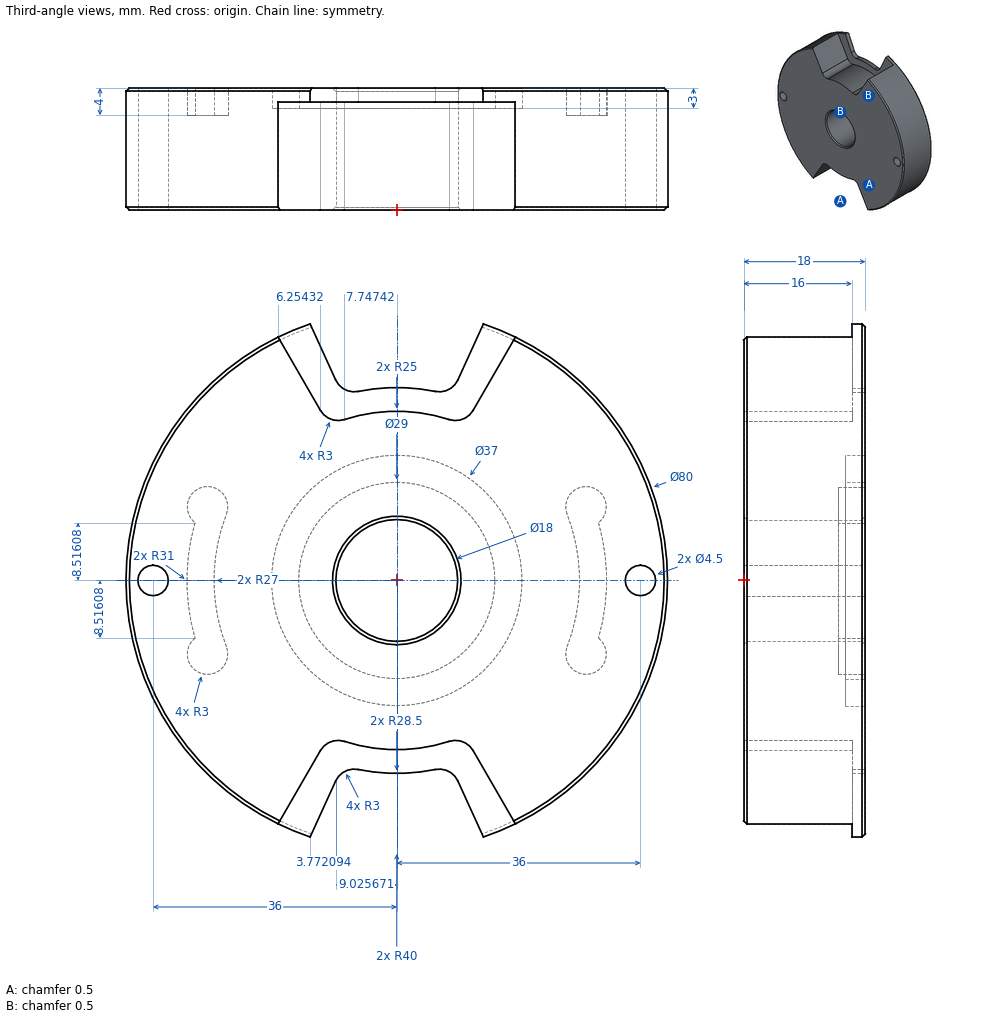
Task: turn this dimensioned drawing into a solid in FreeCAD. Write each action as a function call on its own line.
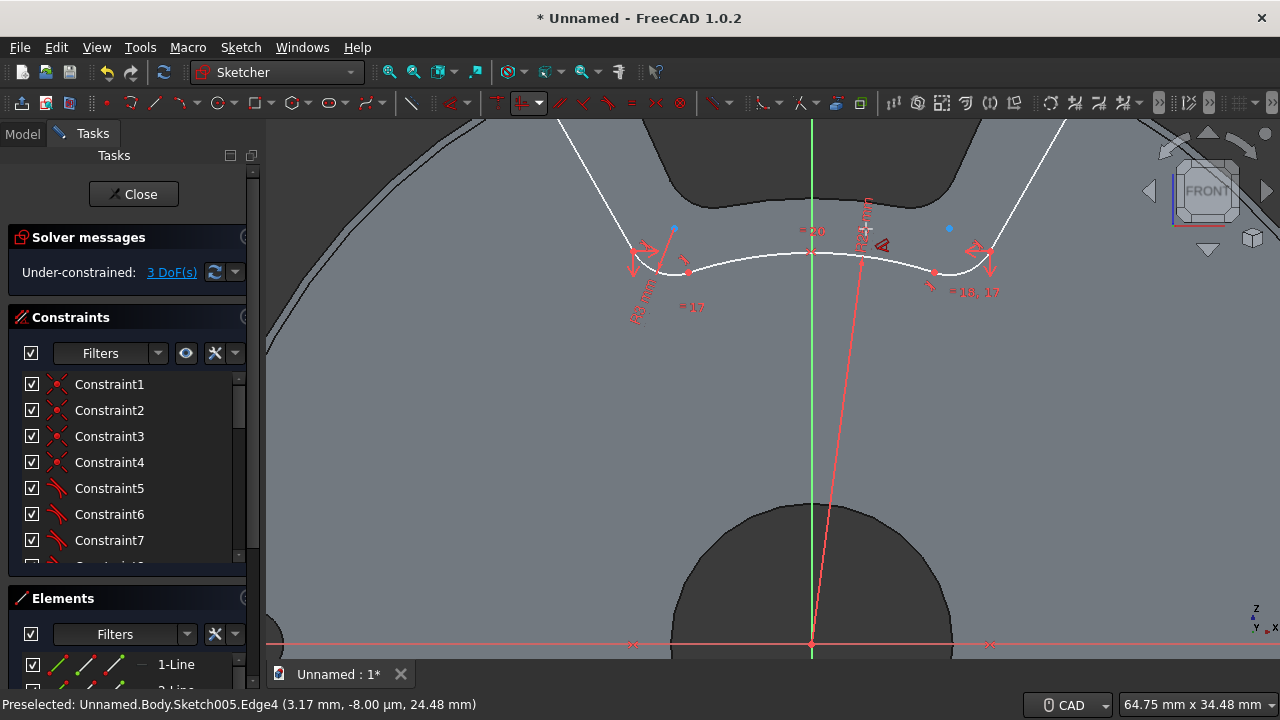
scroll(658, 279, down, 6)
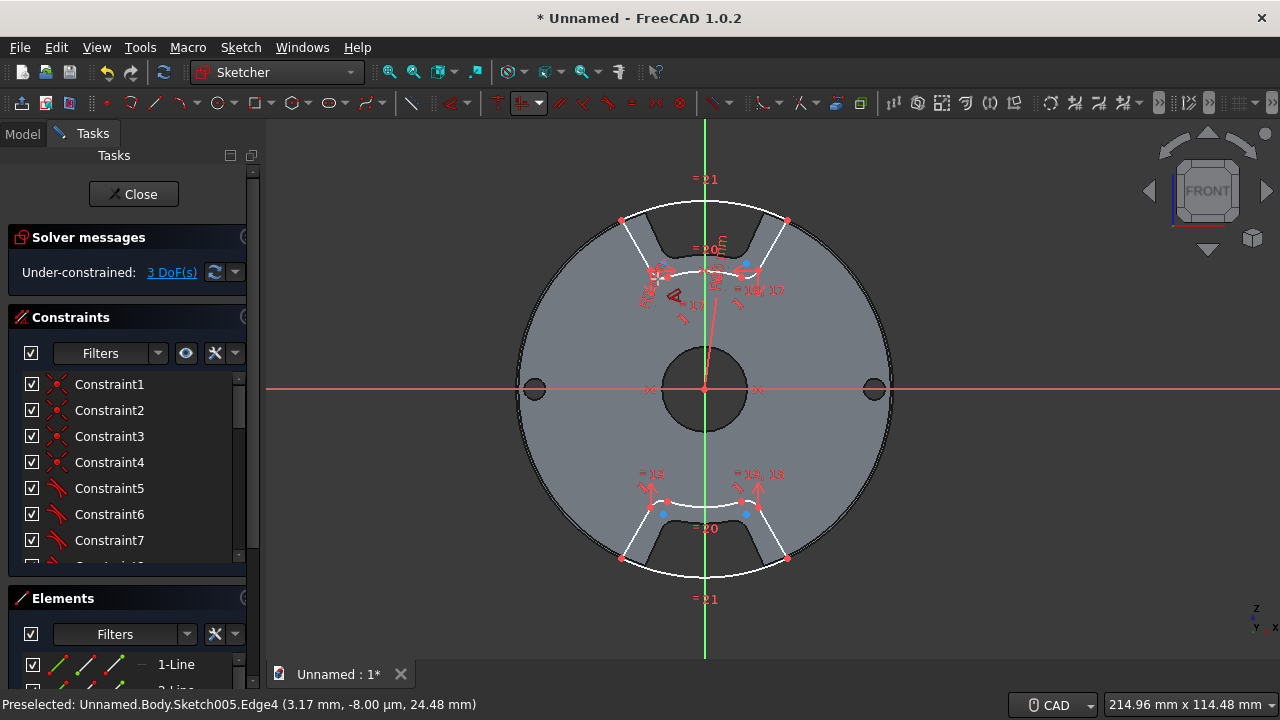
click(739, 204)
click(745, 173)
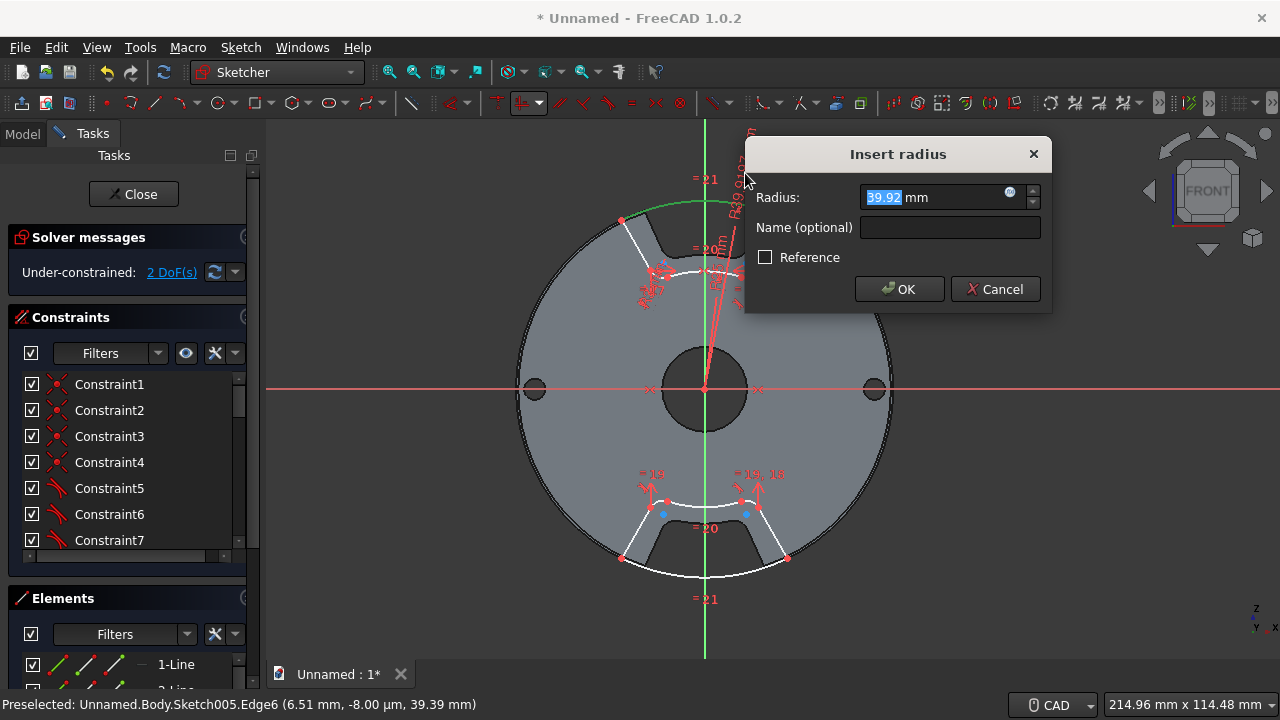
text(40)
key(Return)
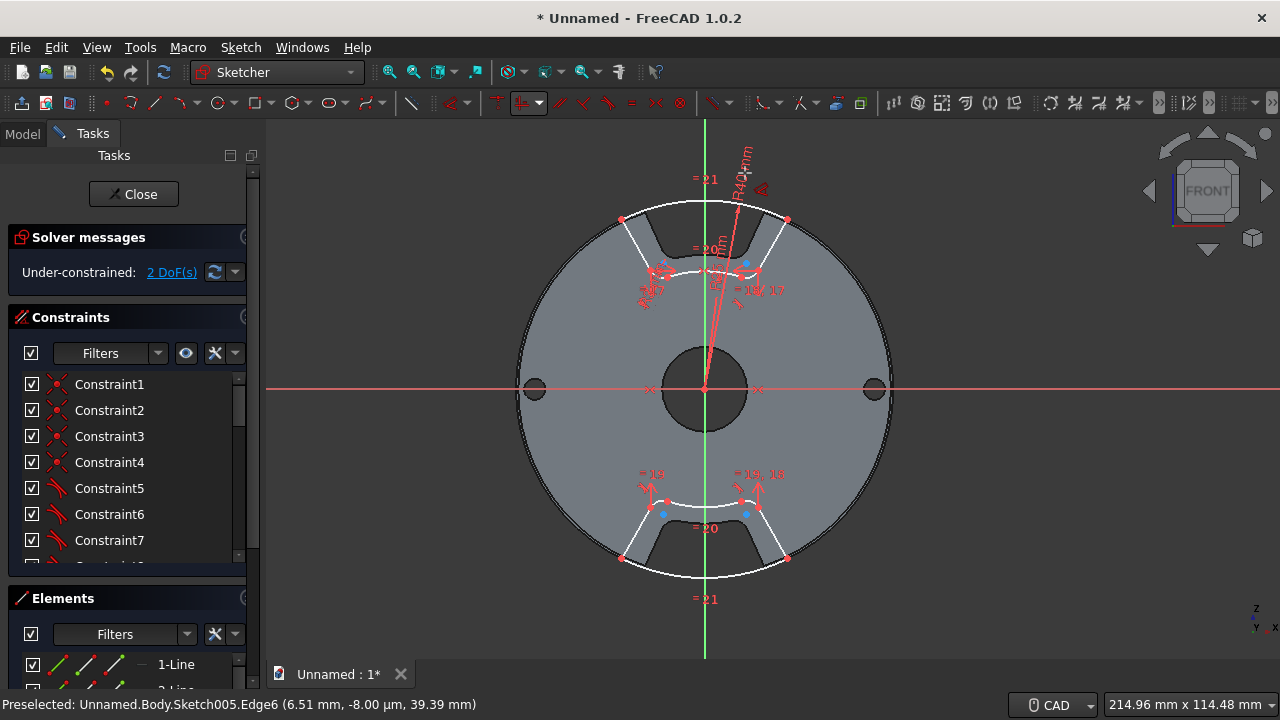
click(668, 277)
click(686, 243)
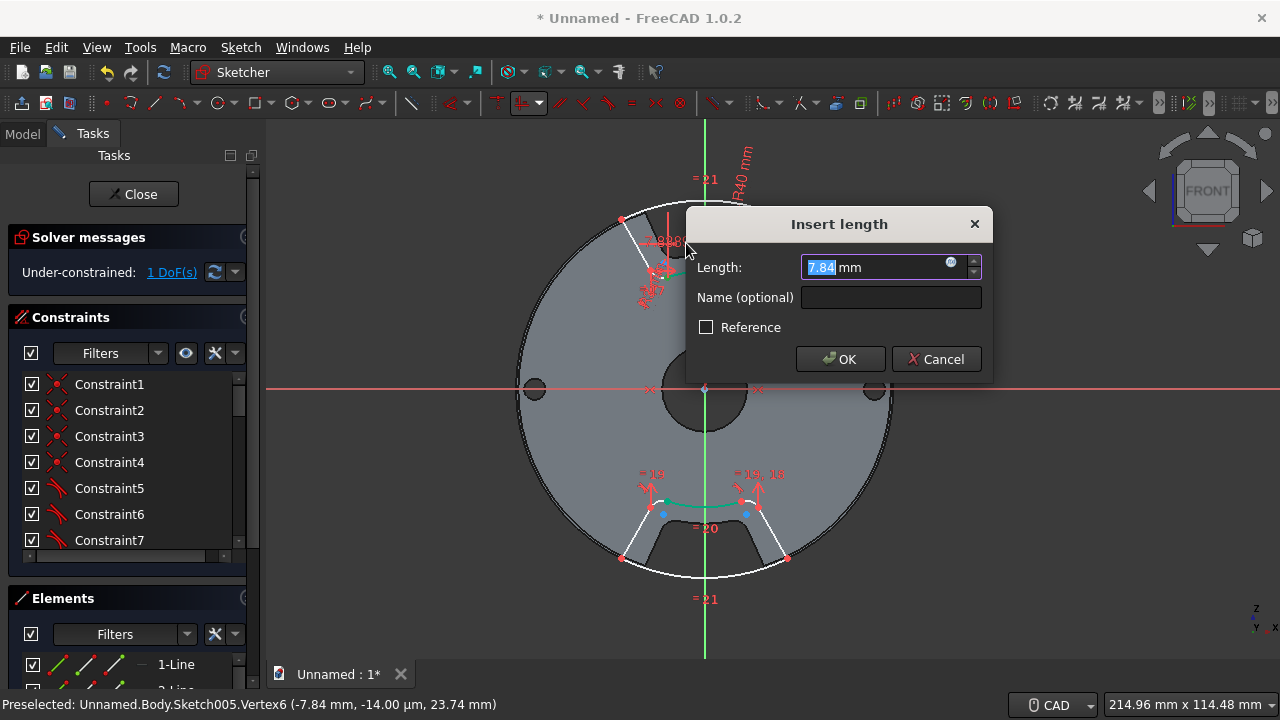
text(7.74742)
key(Return)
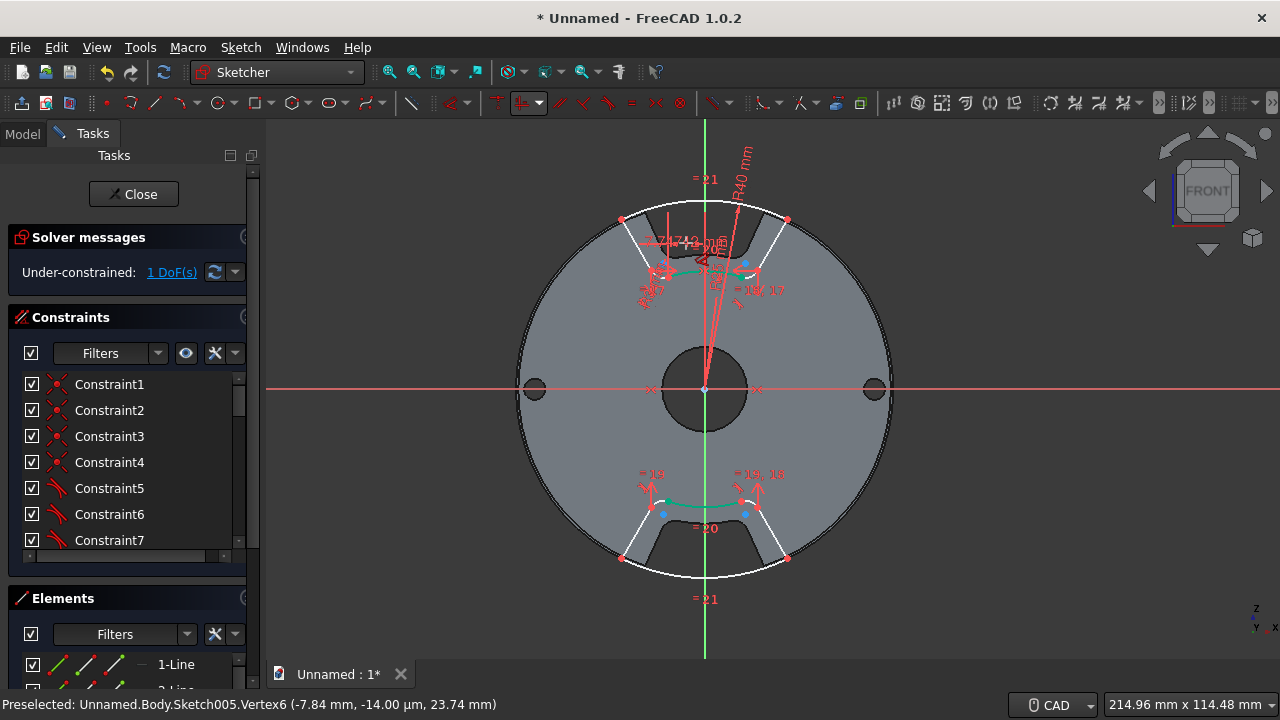
scroll(631, 235, up, 2)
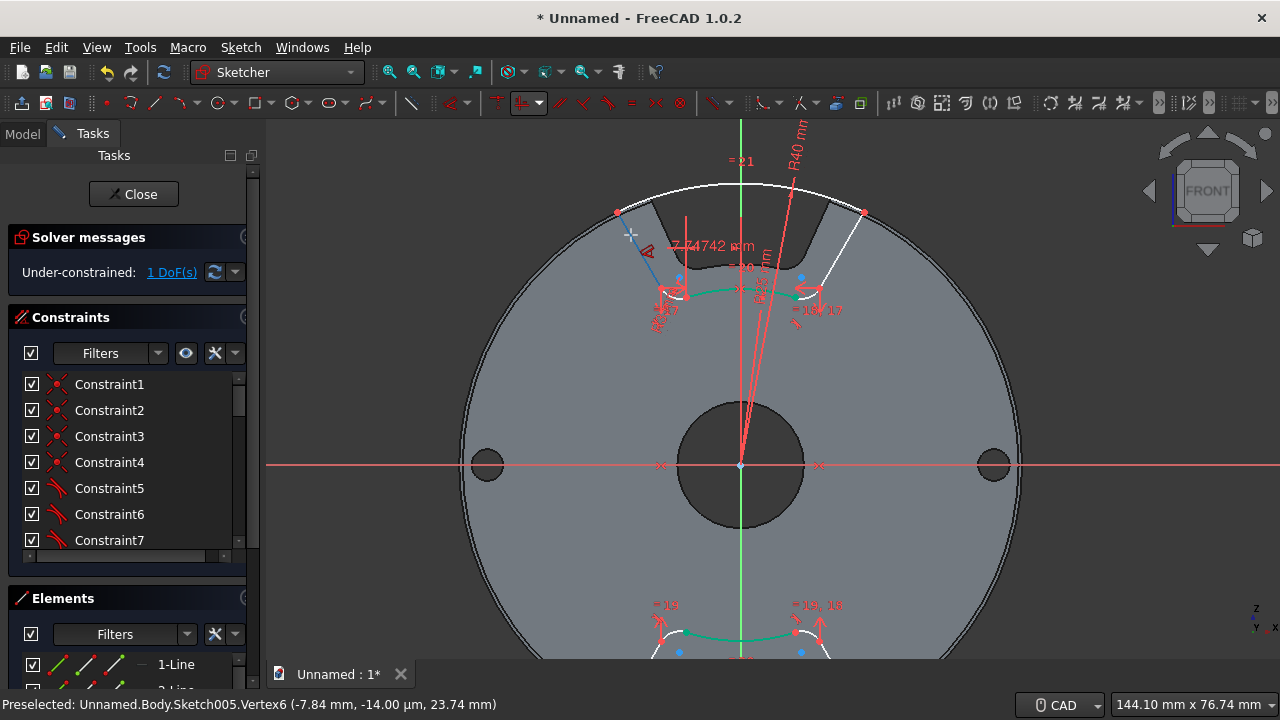
click(630, 235)
click(639, 178)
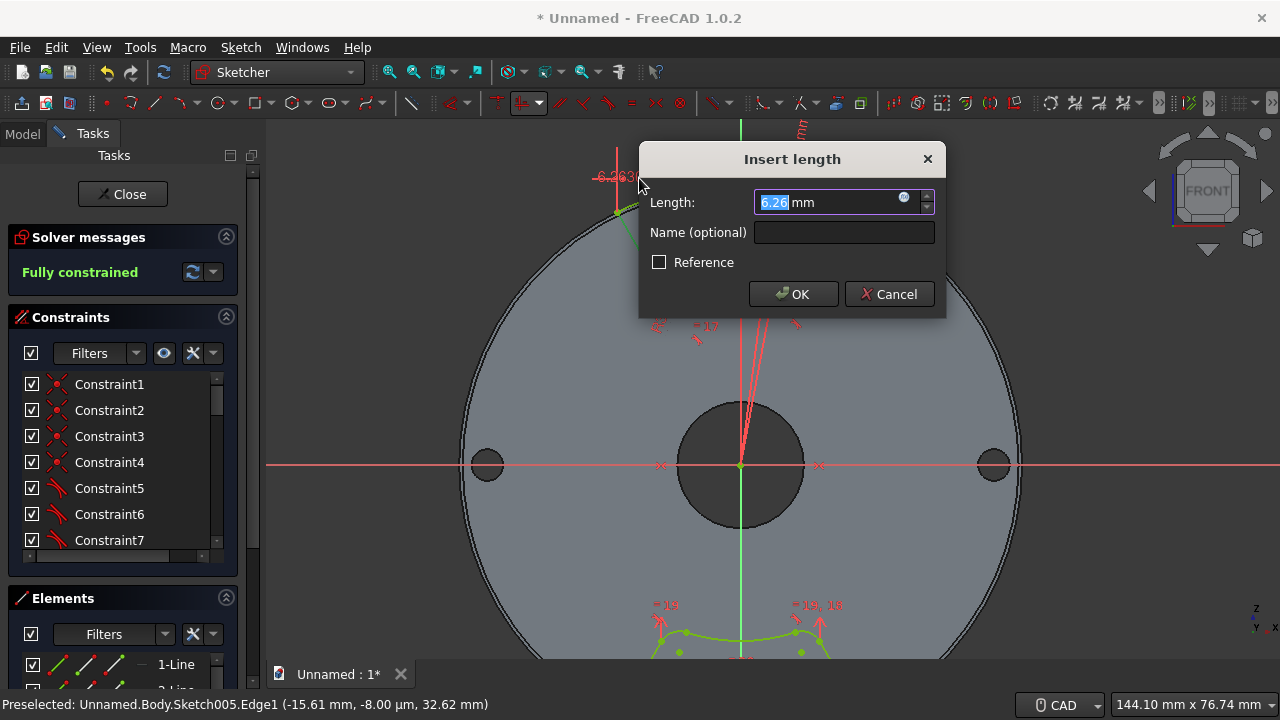
text(6.25432)
key(Return)
key(Escape)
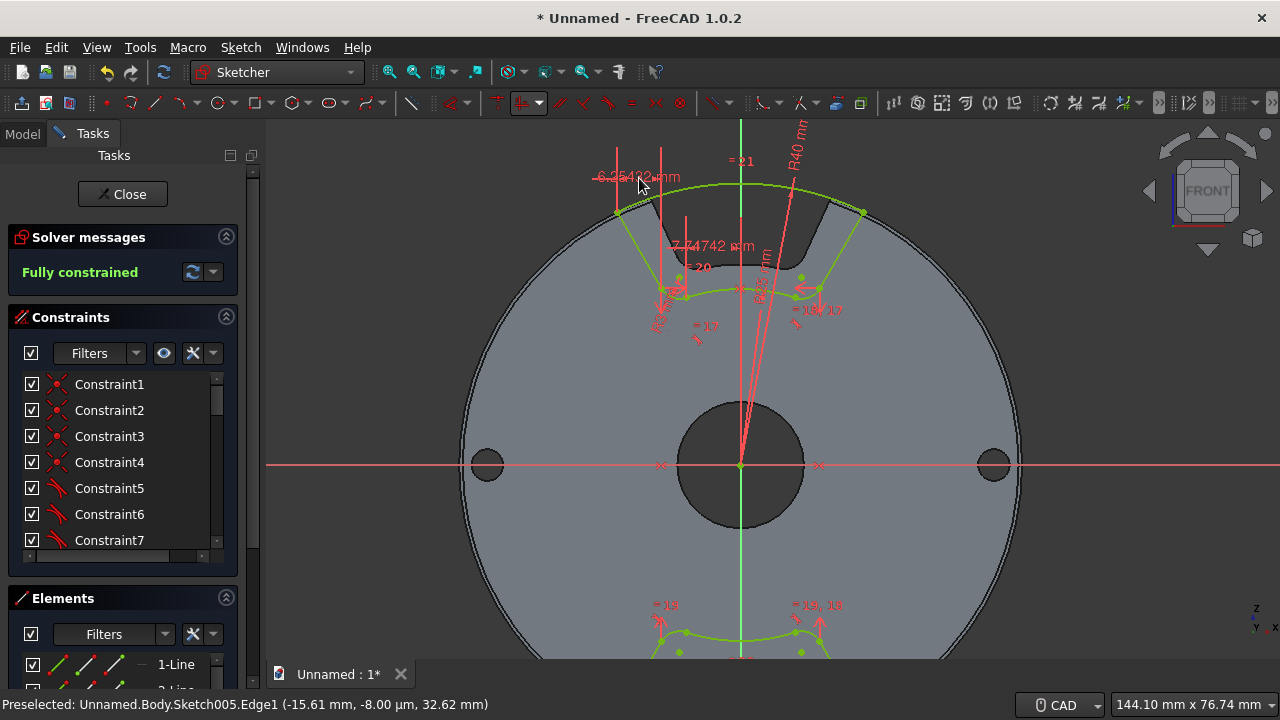
click(123, 194)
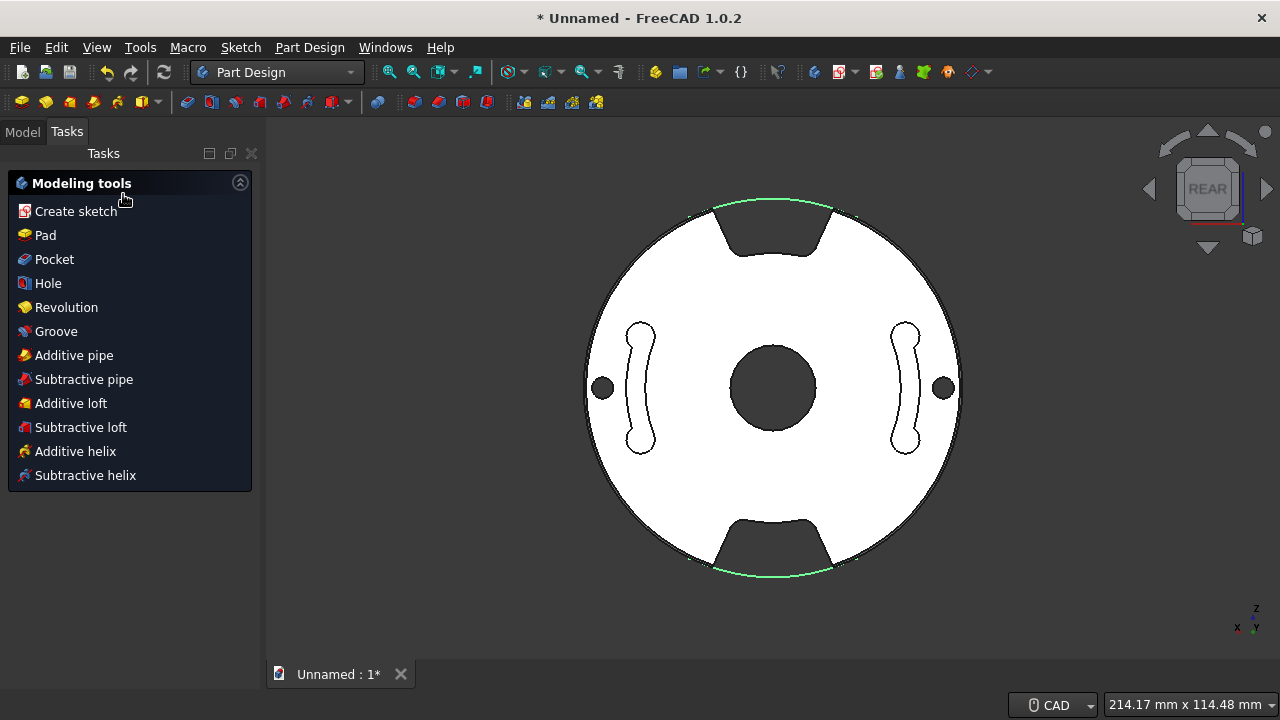
click(188, 102)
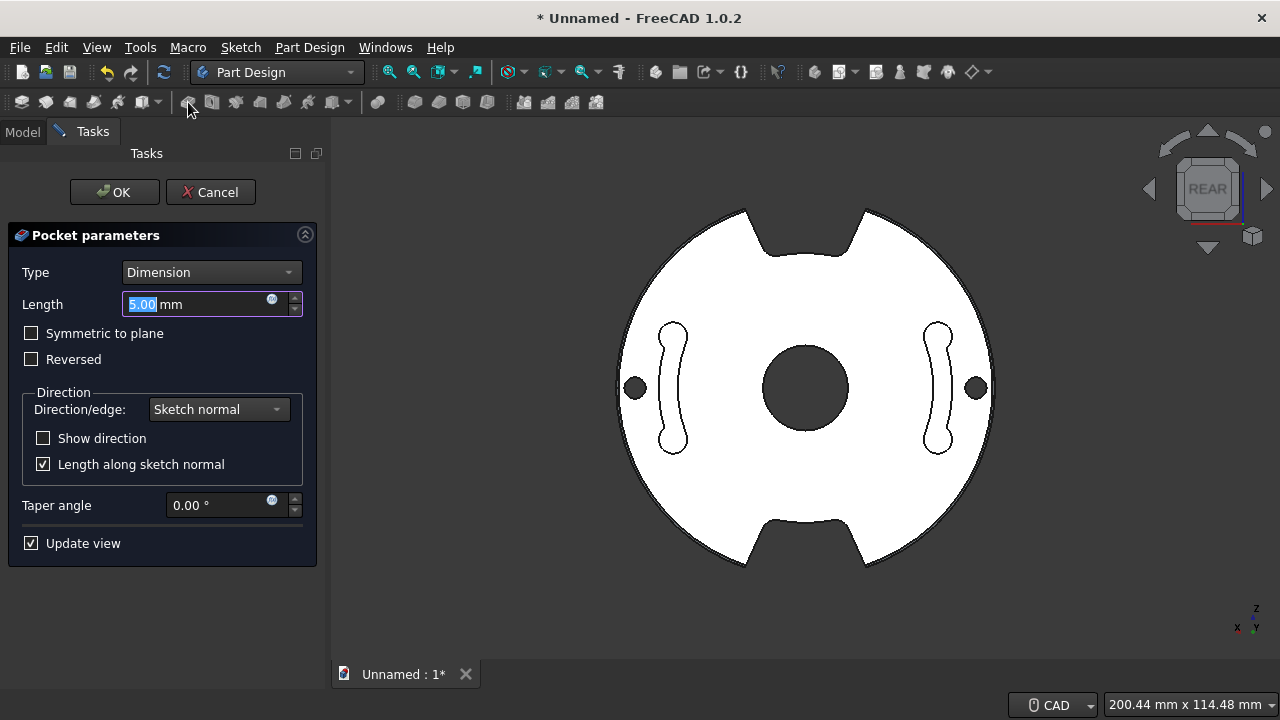
text(16)
key(Tab)